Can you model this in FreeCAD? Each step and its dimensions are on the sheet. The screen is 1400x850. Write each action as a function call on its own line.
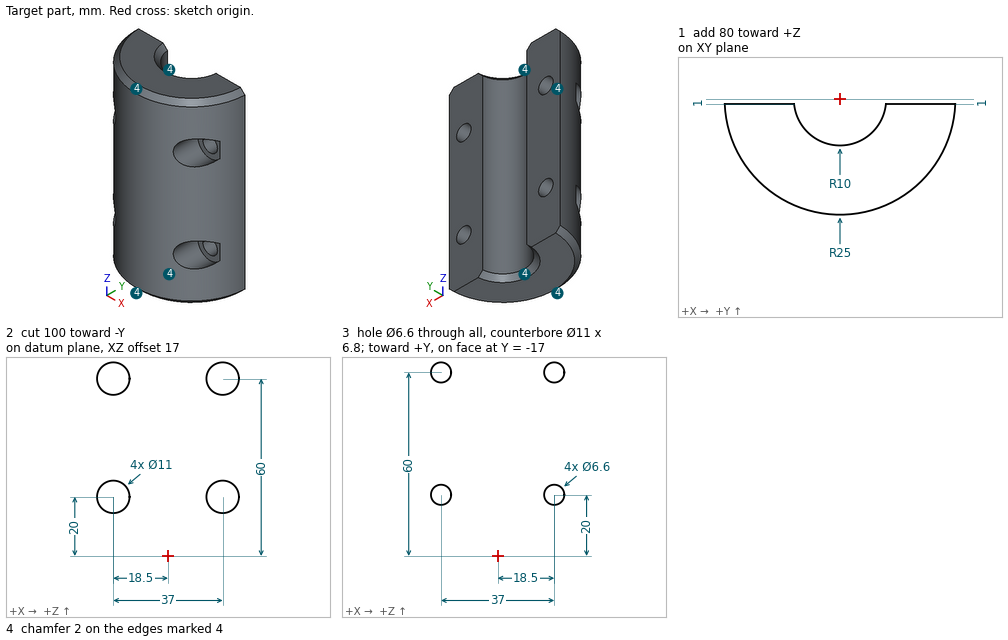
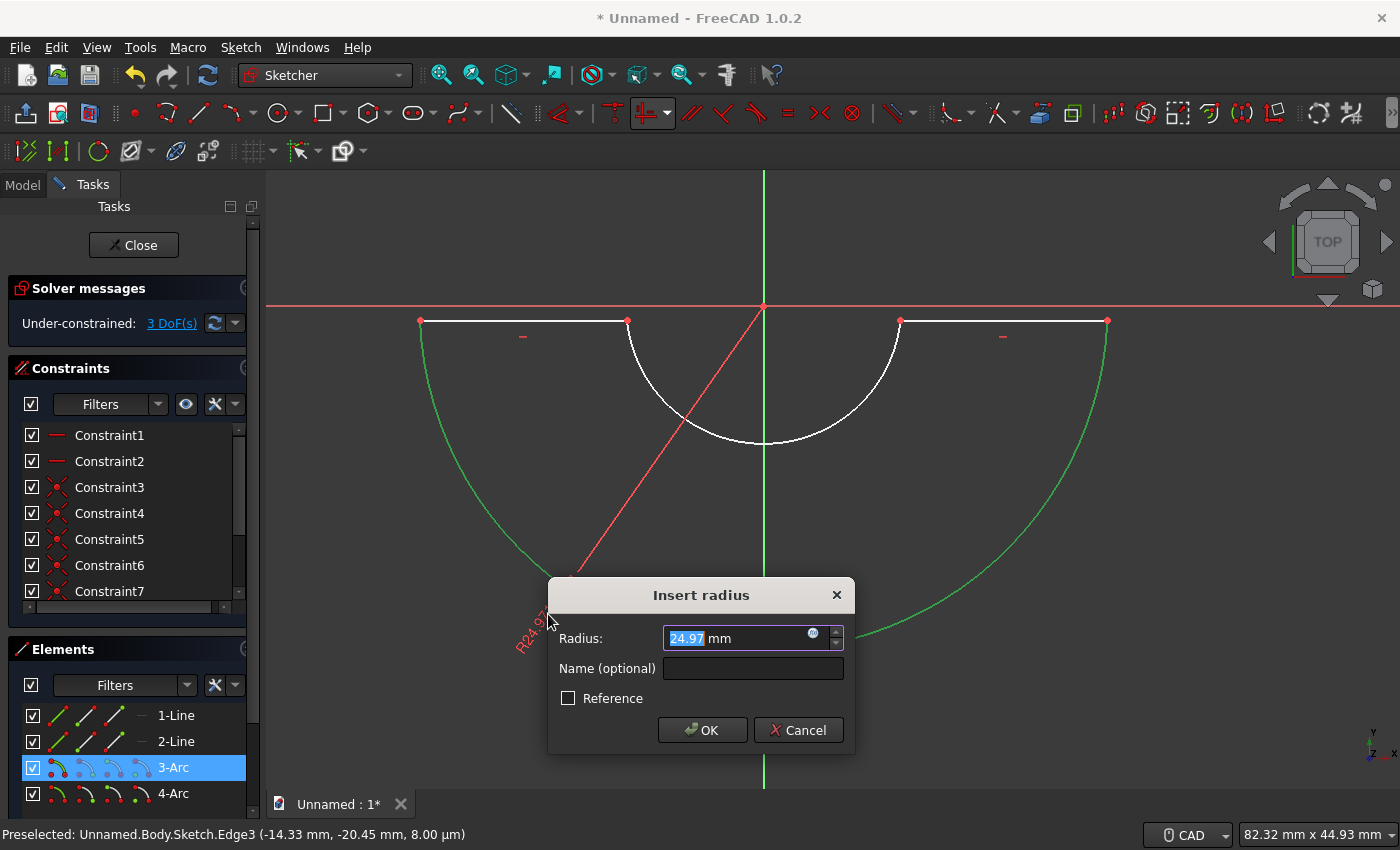
text(25)
key(Return)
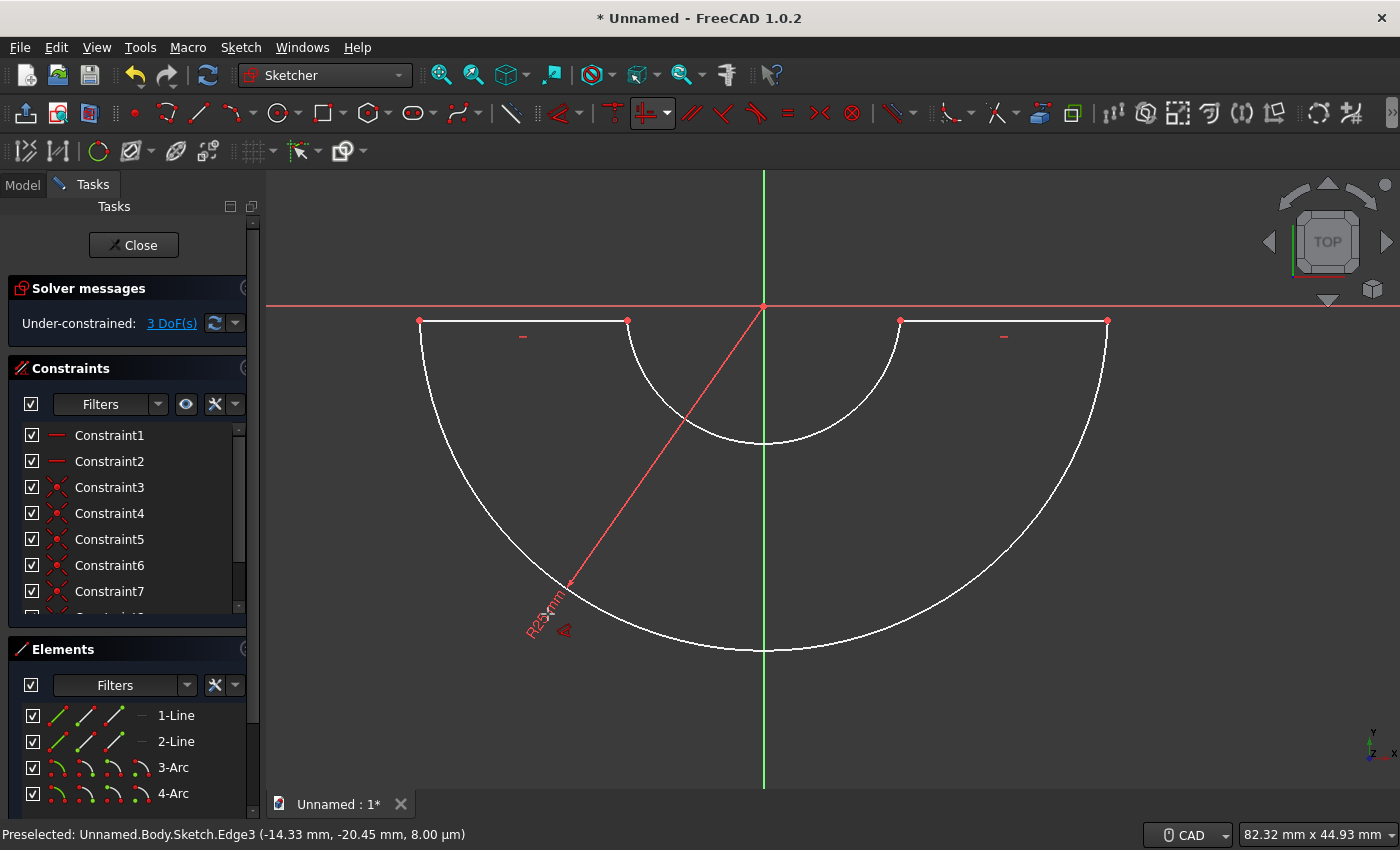
click(688, 421)
click(670, 448)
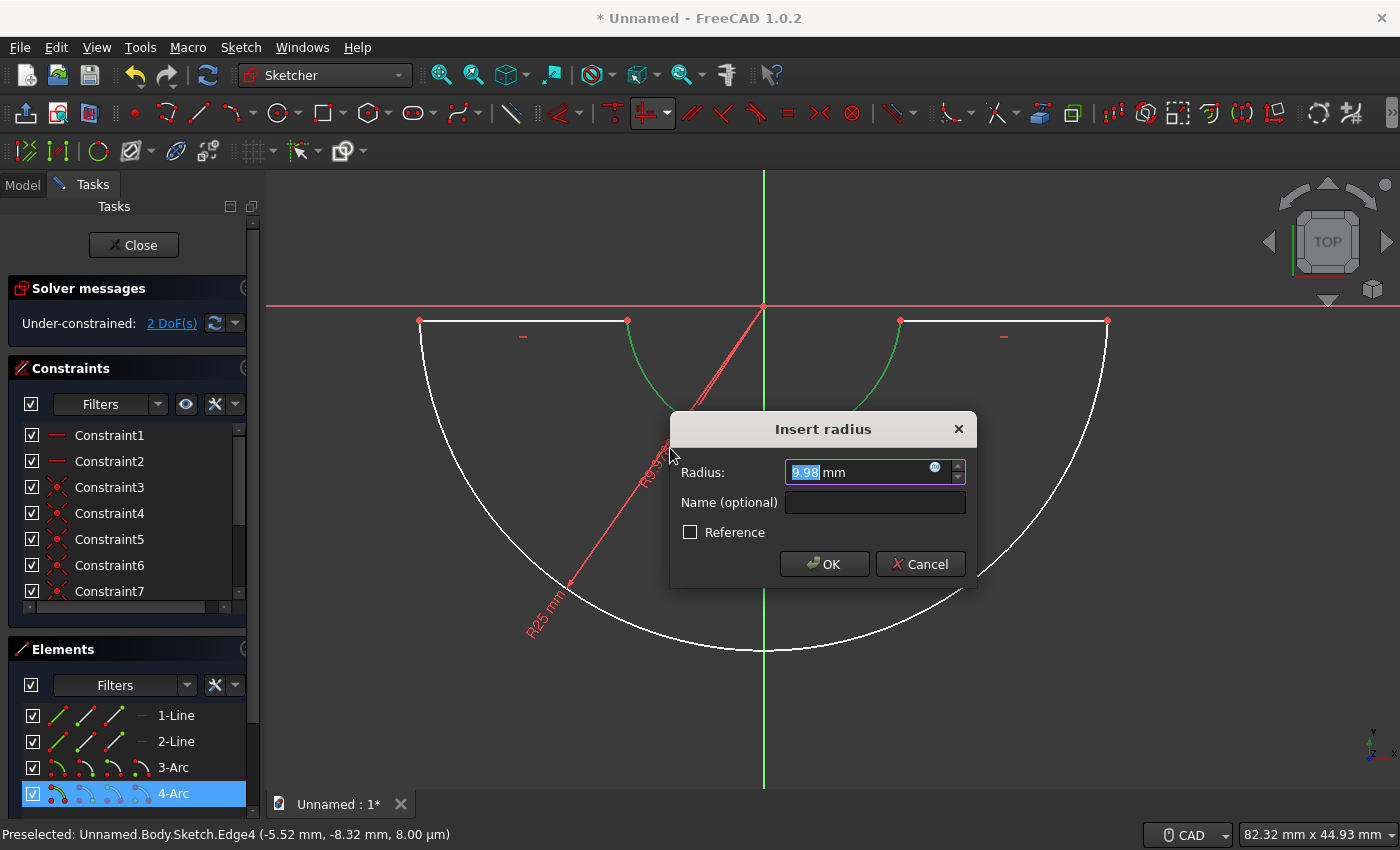
text(10)
key(Return)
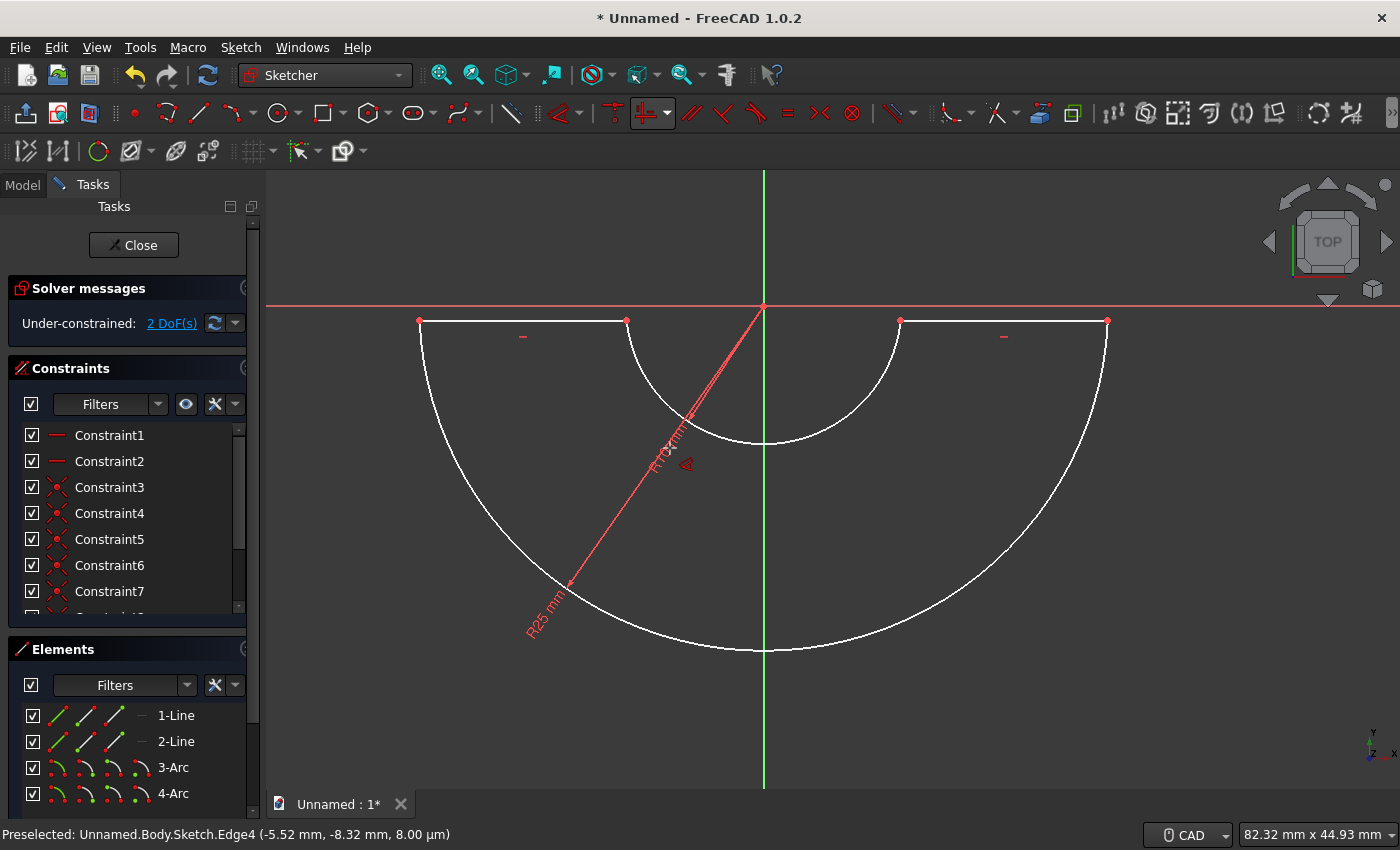
scroll(627, 321, up, 6)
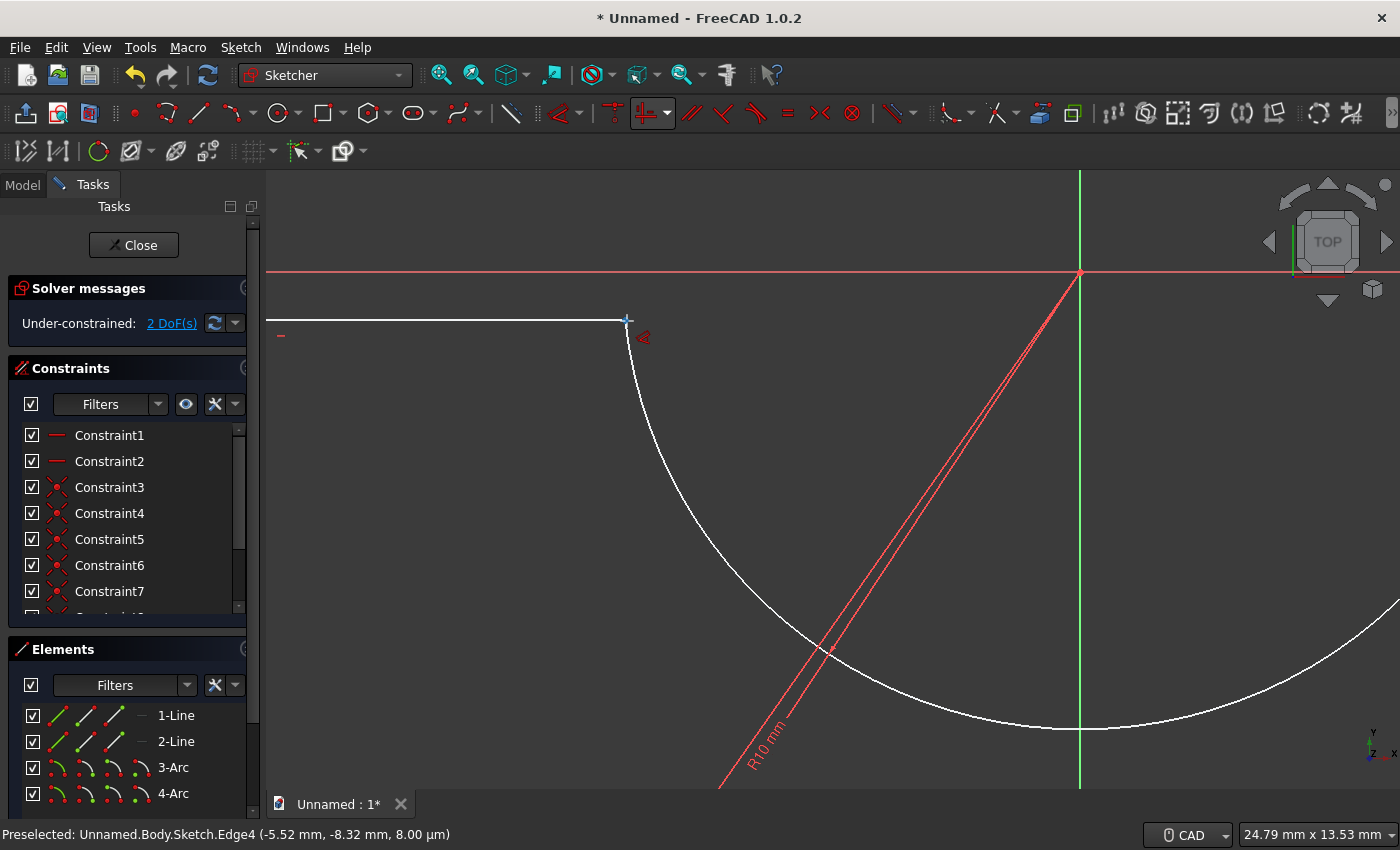
click(625, 320)
click(591, 296)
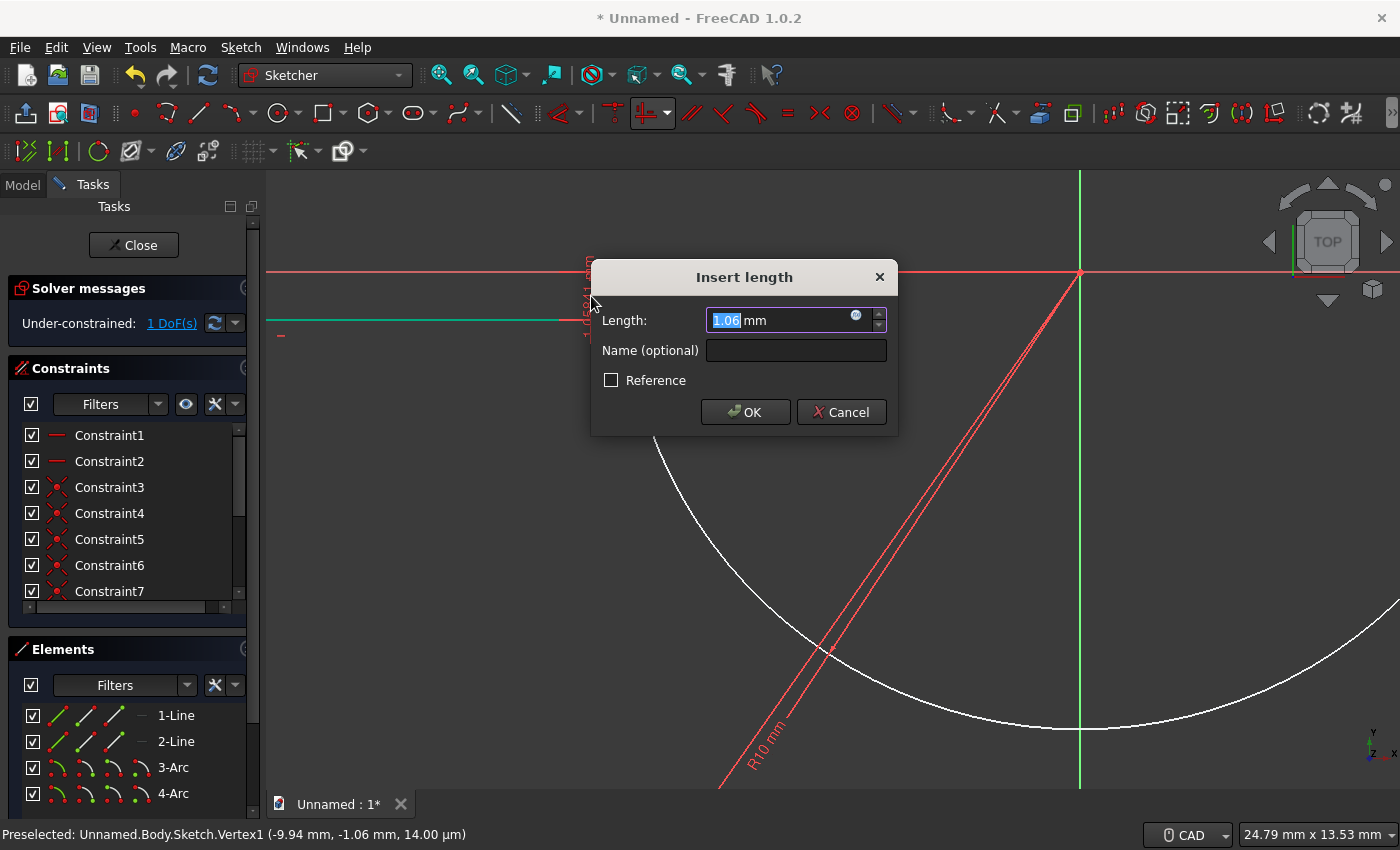
text(1)
key(Return)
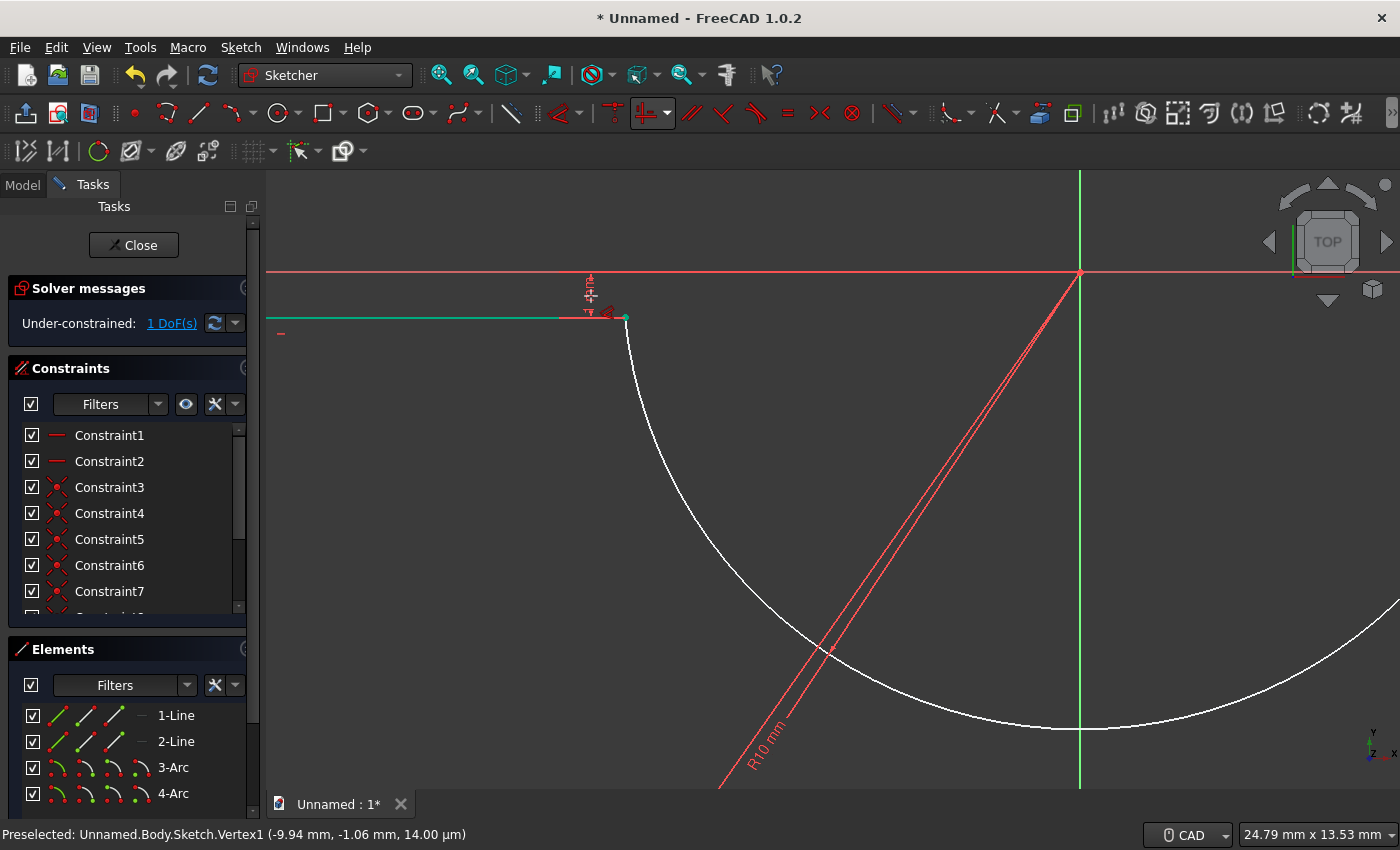
scroll(628, 323, down, 6)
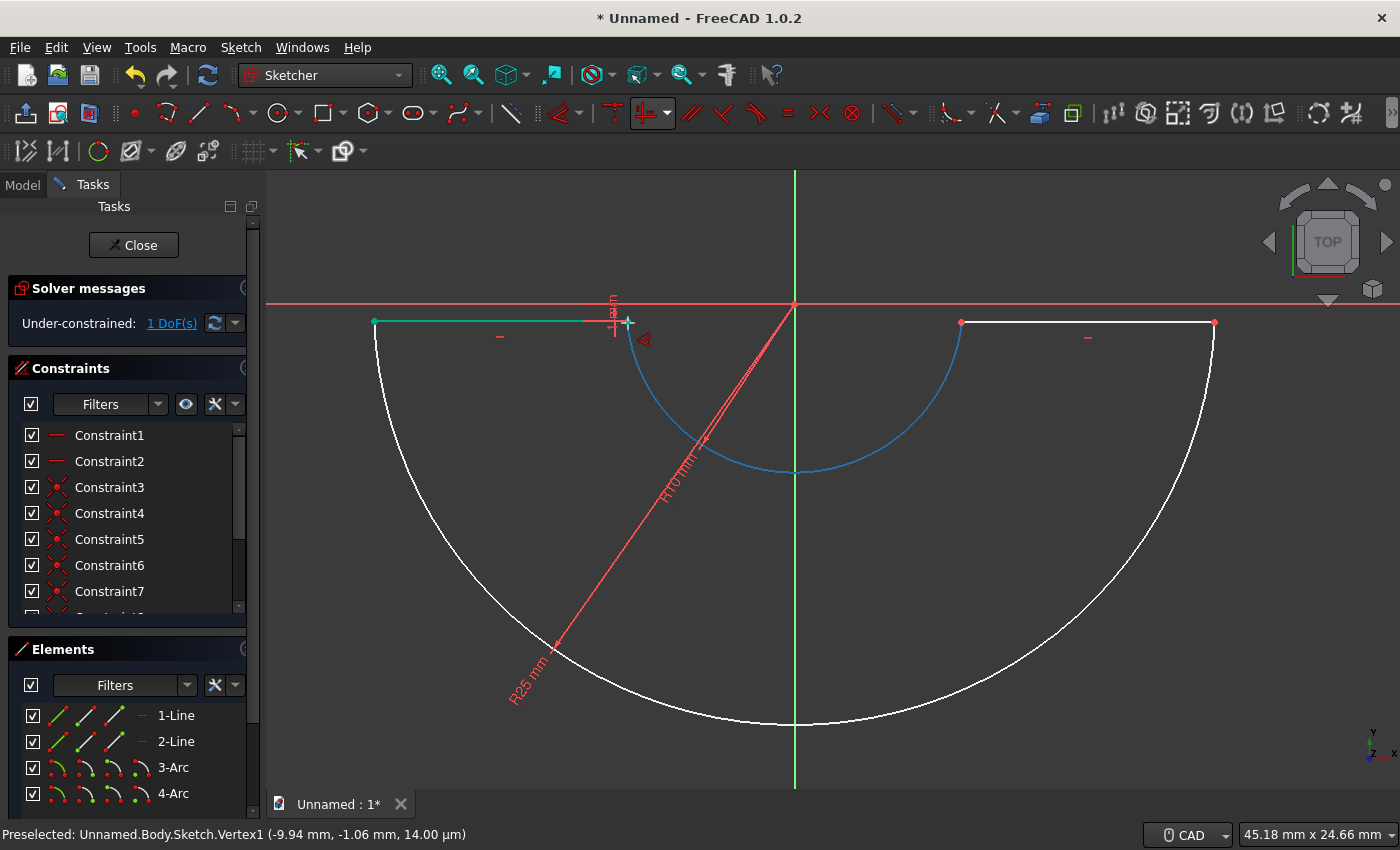
scroll(1108, 322, up, 6)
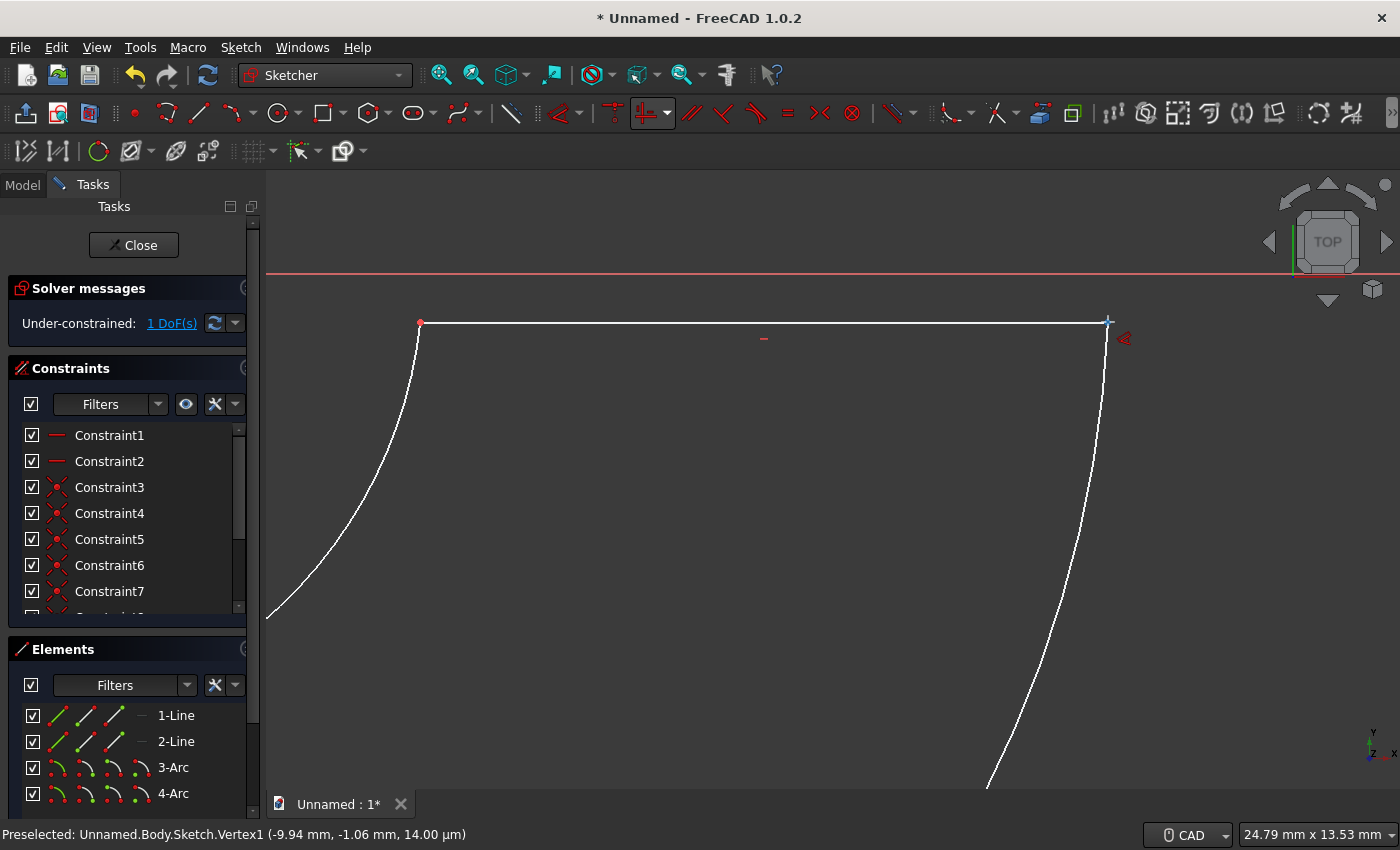
click(1108, 323)
click(1142, 299)